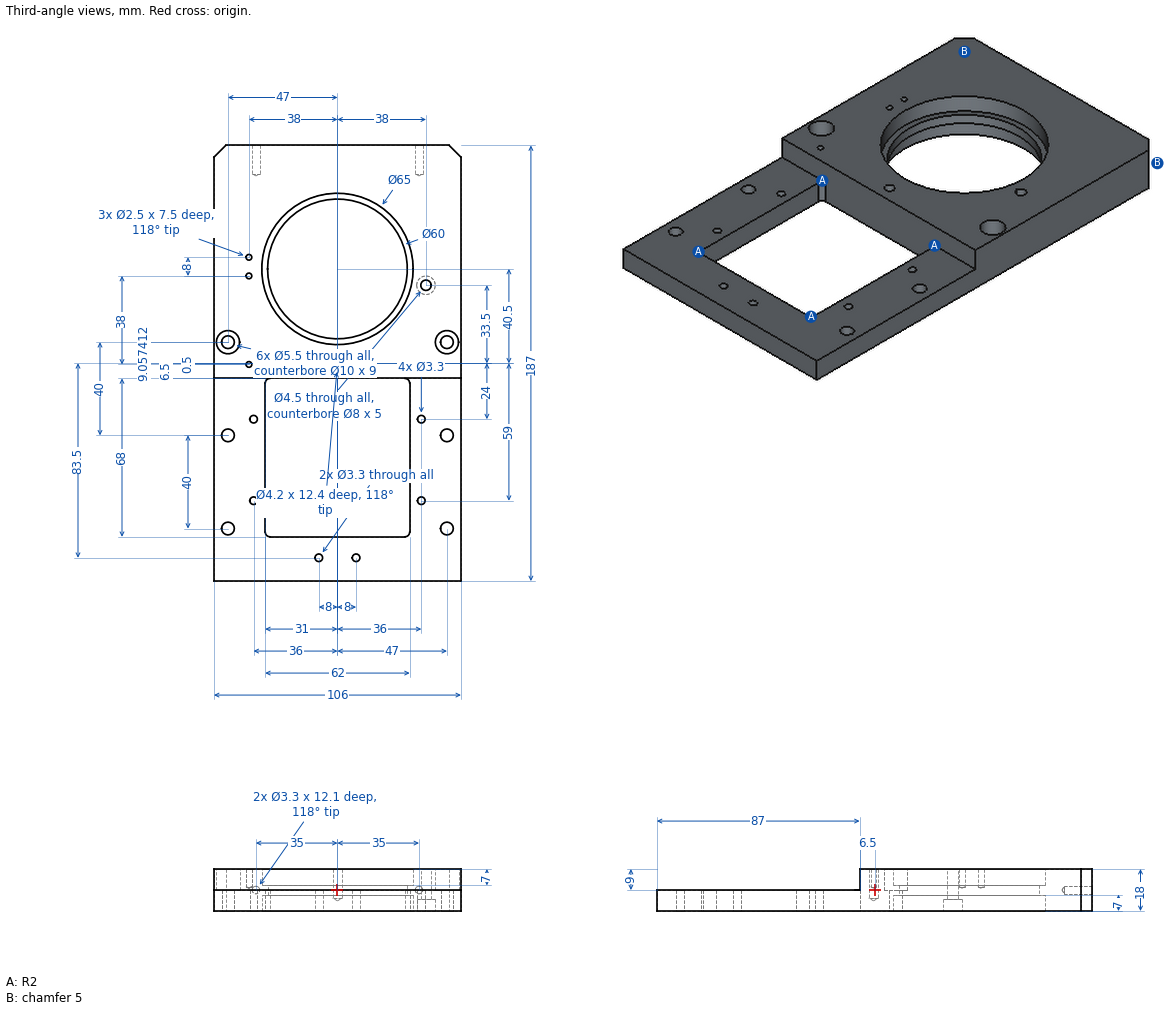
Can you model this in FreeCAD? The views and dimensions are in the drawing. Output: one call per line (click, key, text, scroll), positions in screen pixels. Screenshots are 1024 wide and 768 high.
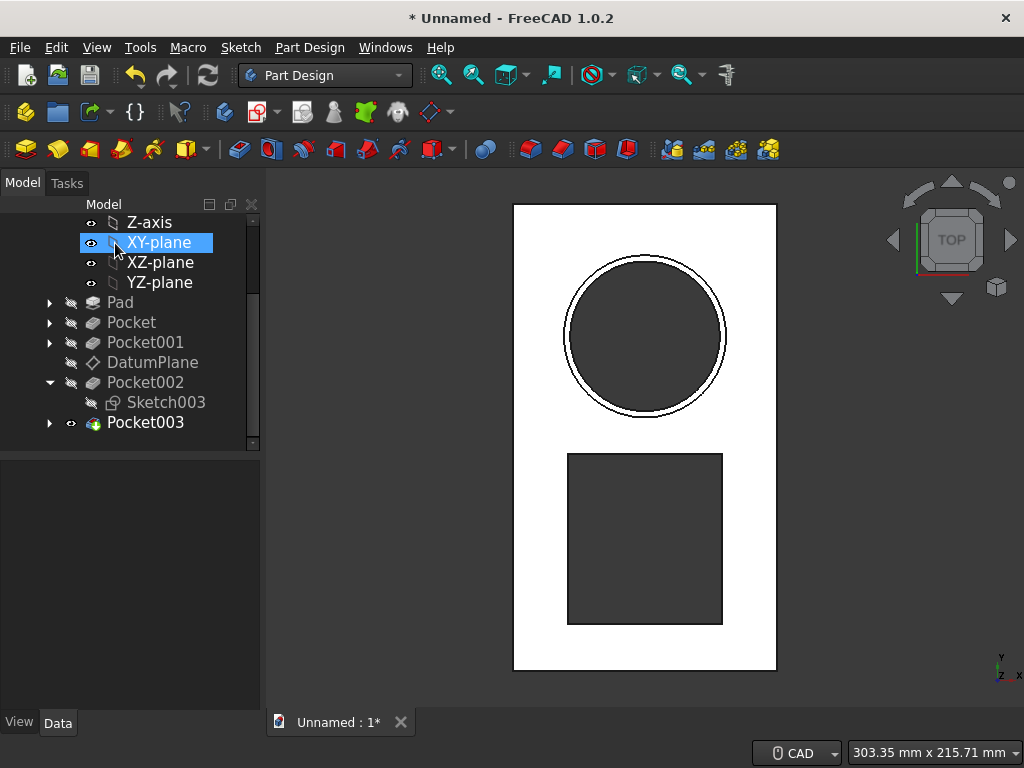
key(0)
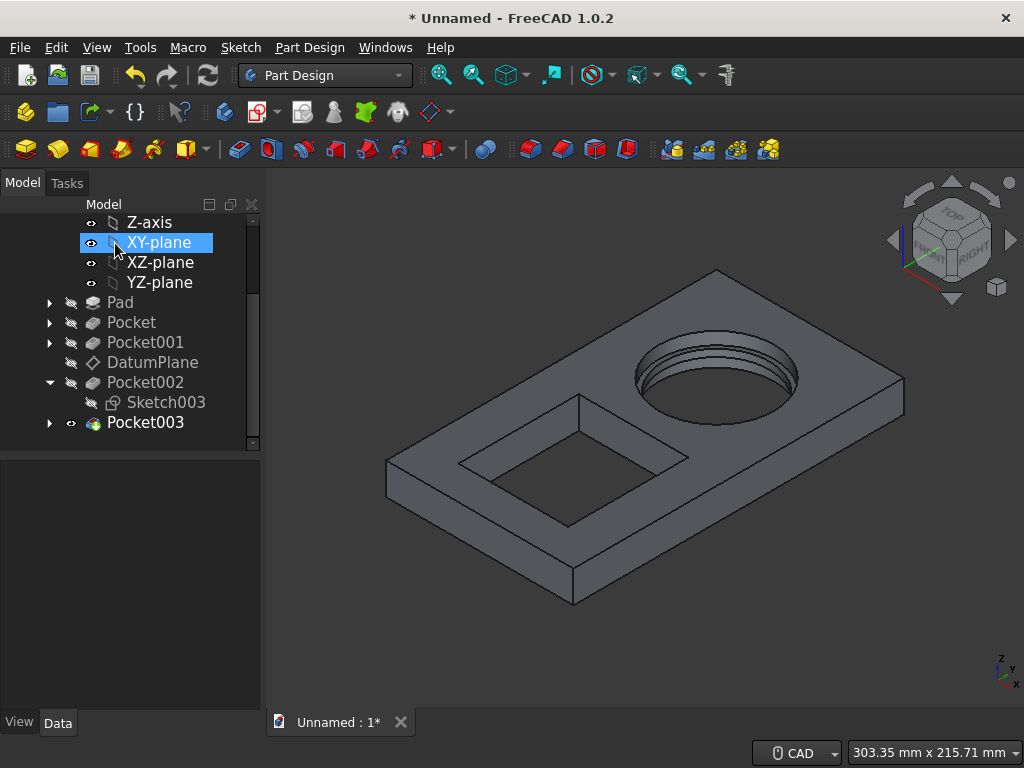
key(1)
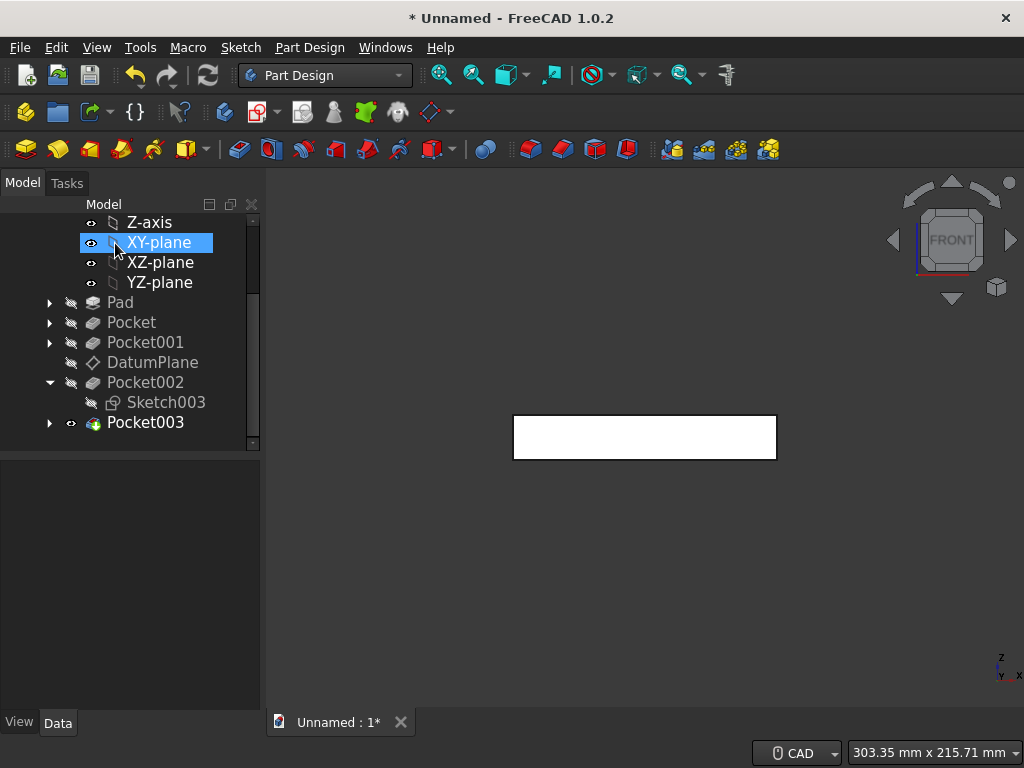
click(442, 76)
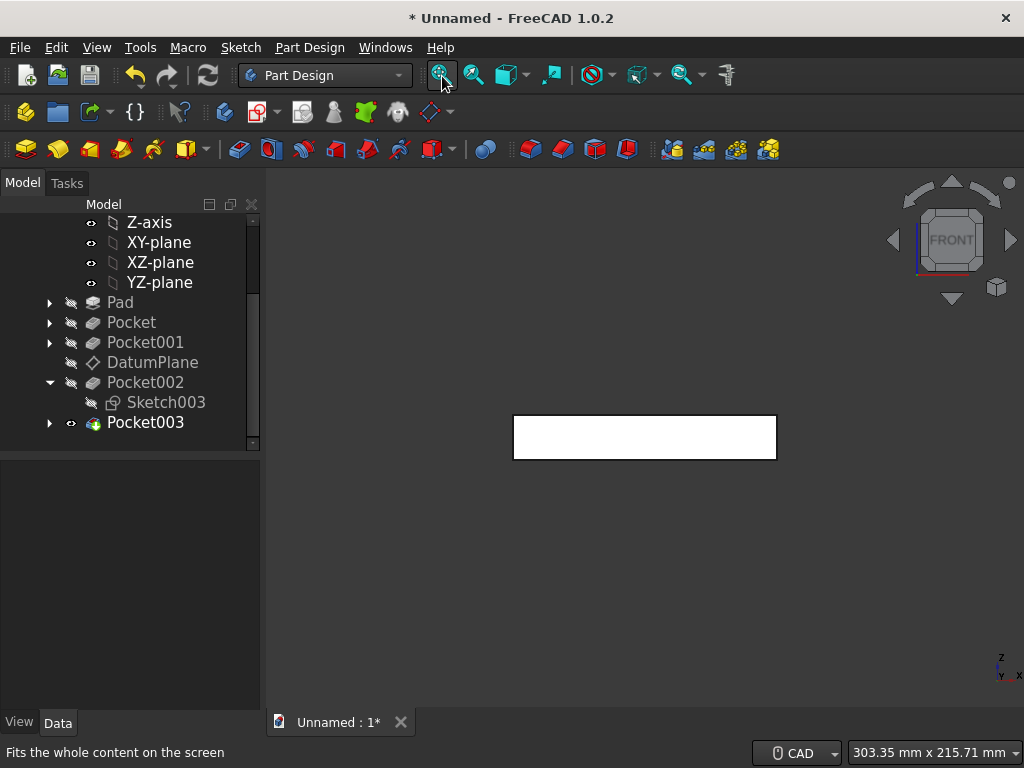
key(3)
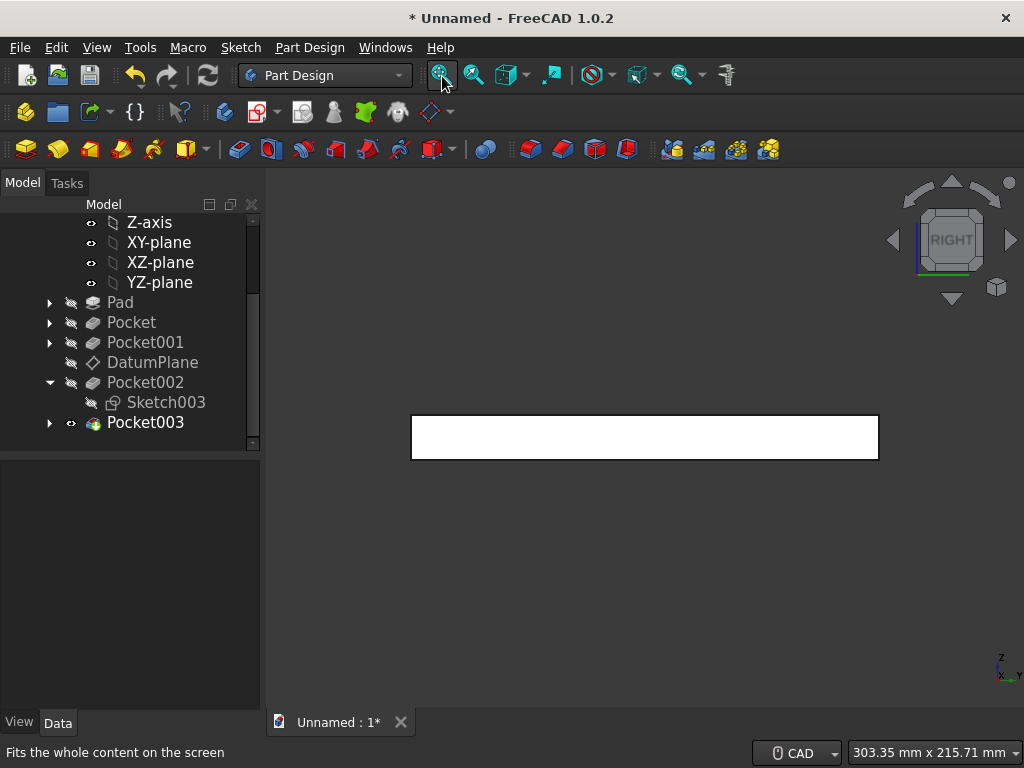
key(5)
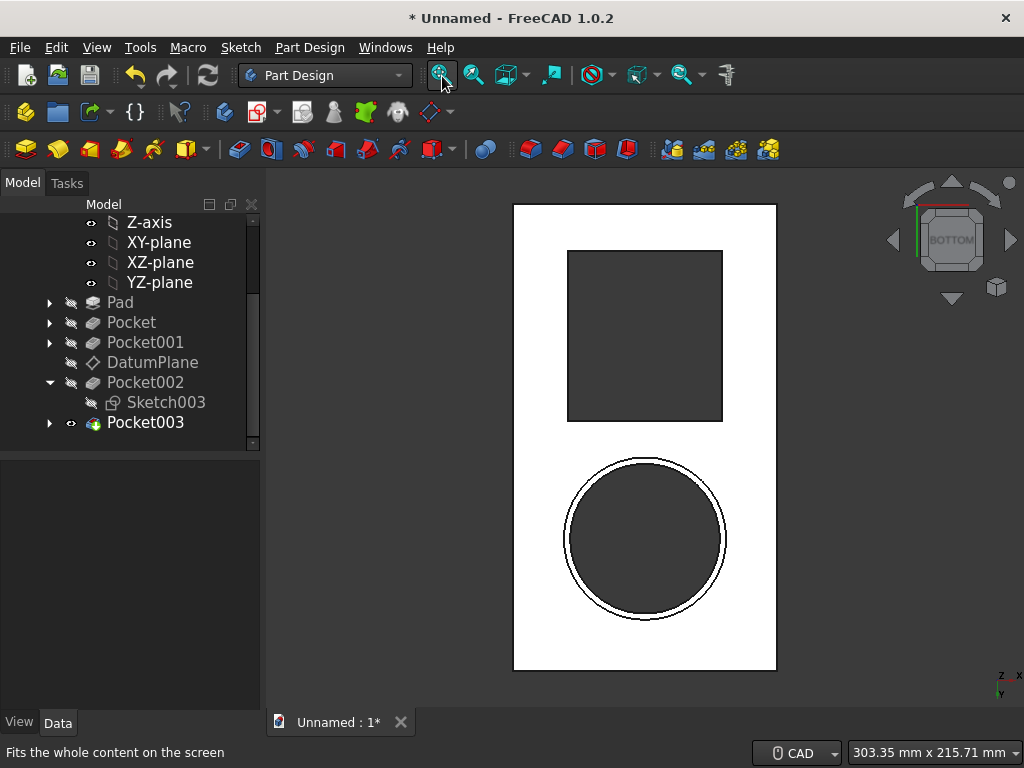
key(4)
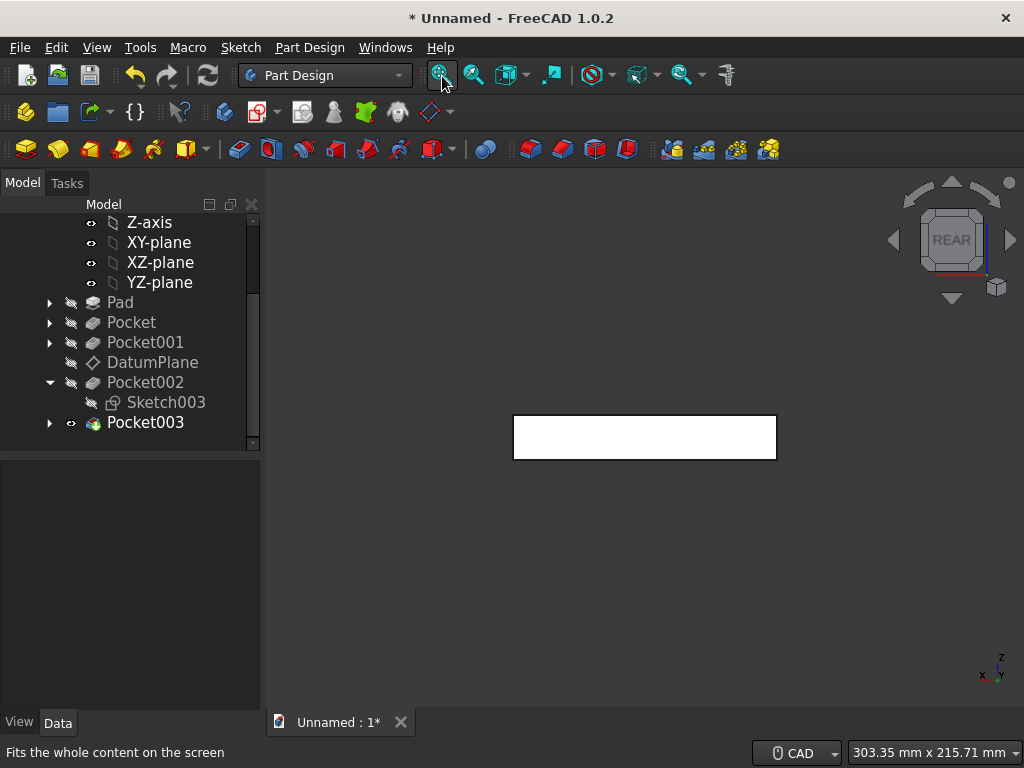
click(442, 76)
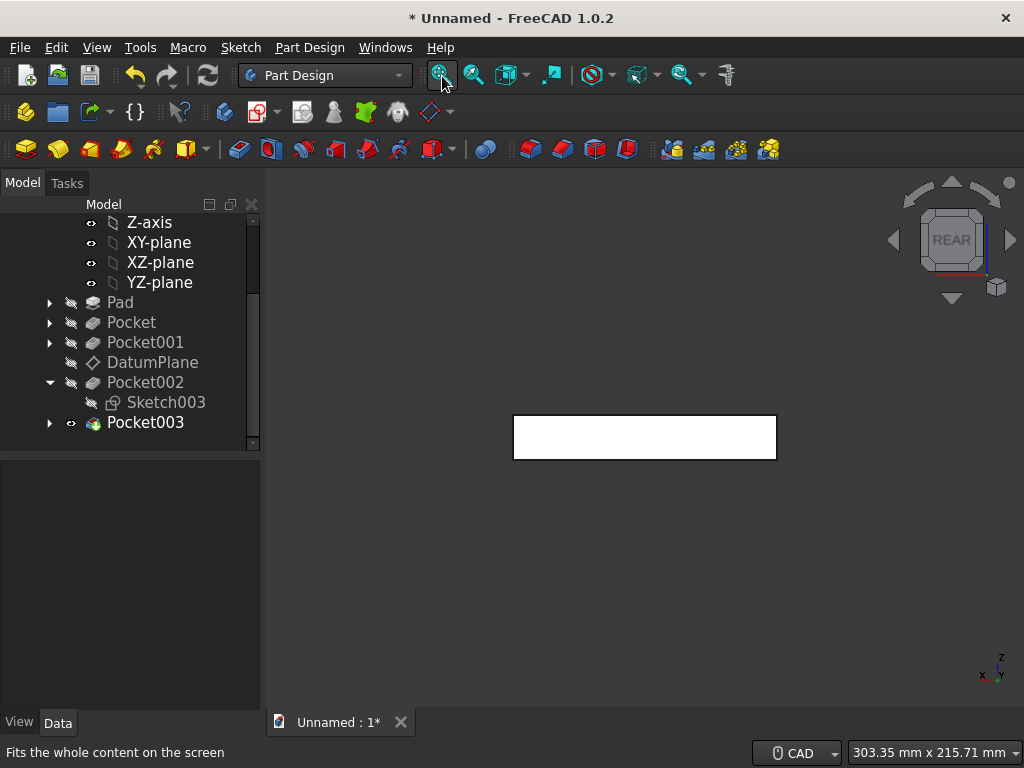
key(6)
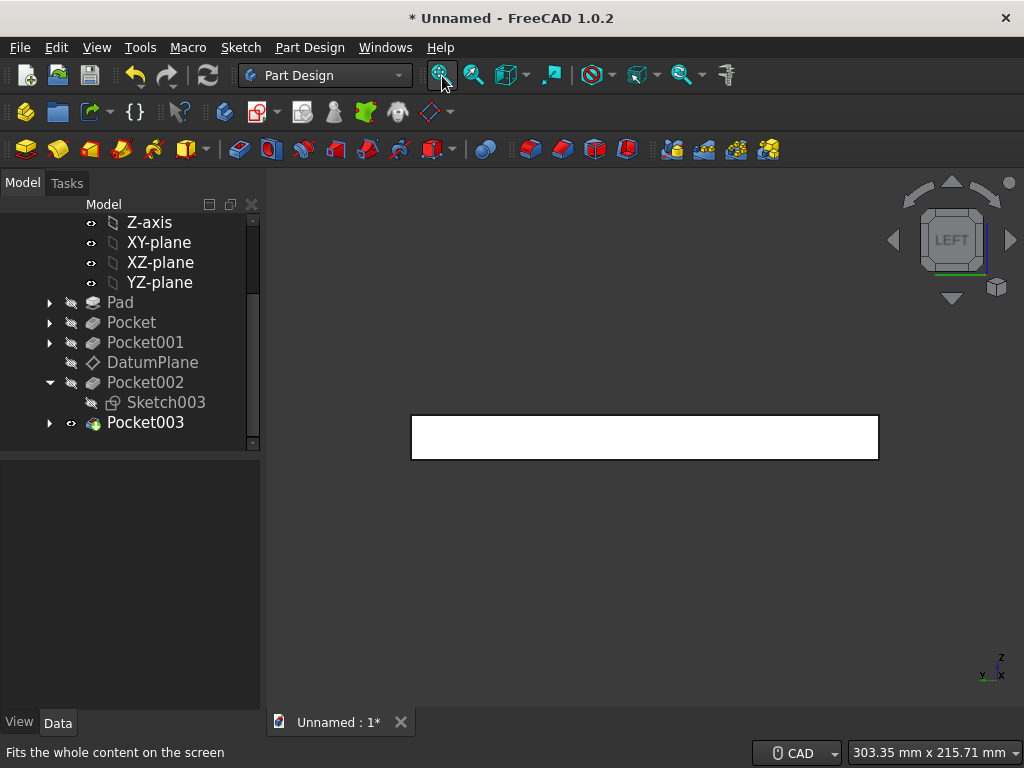
key(v)
key(3)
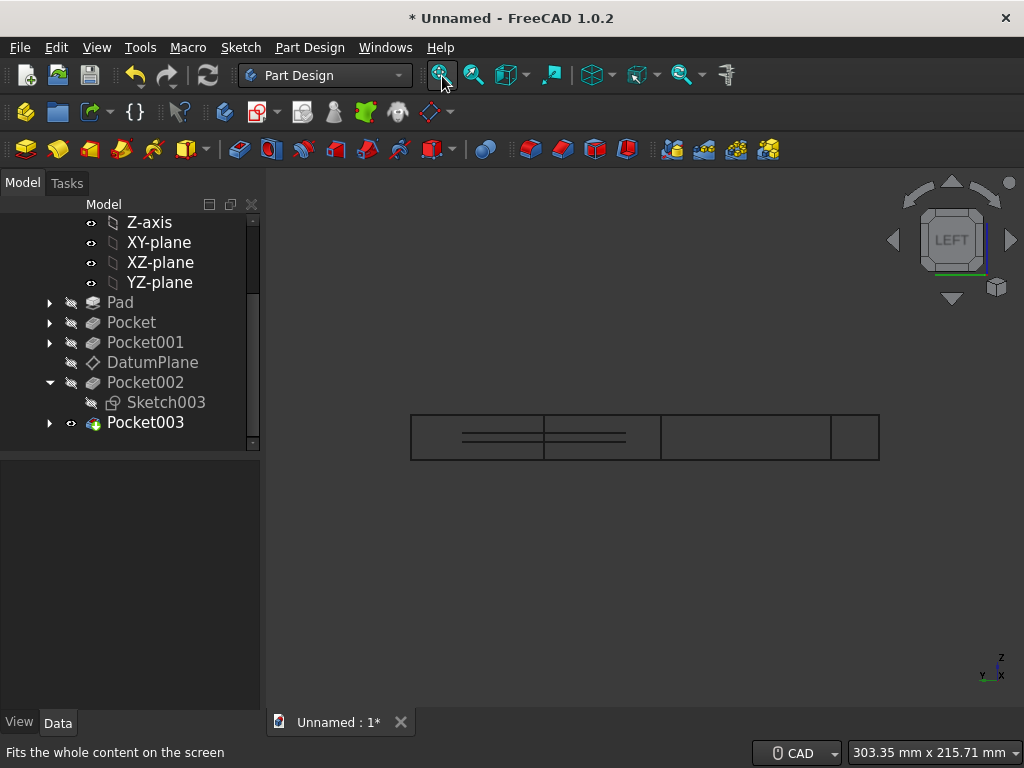
key(0)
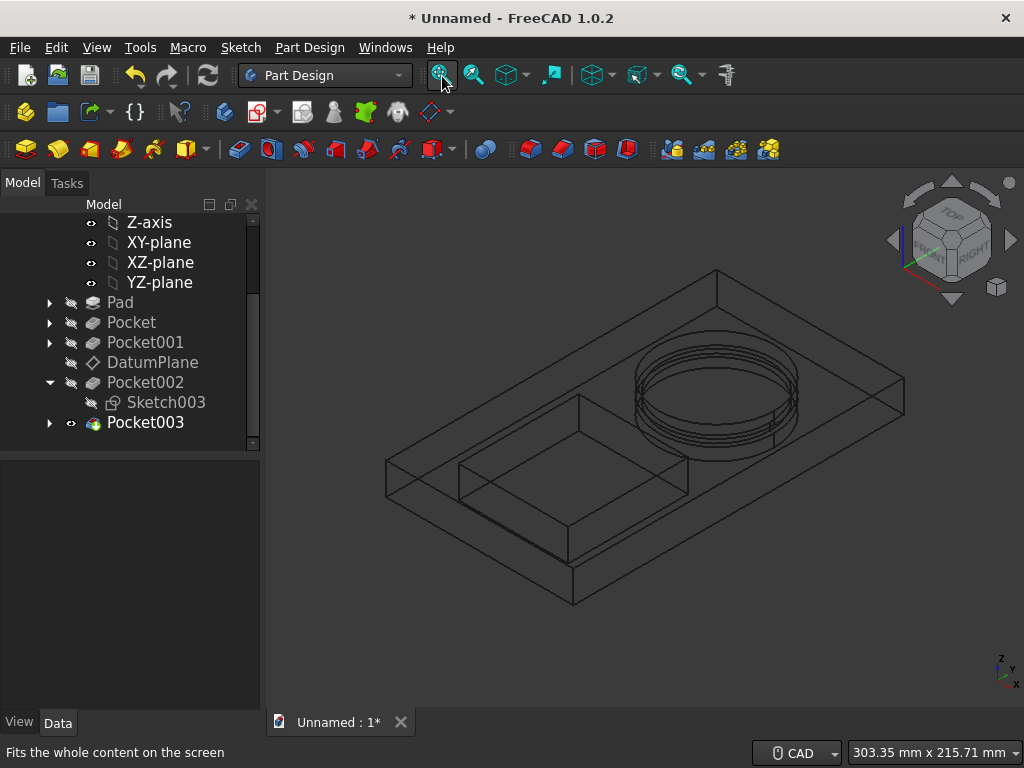
click(459, 481)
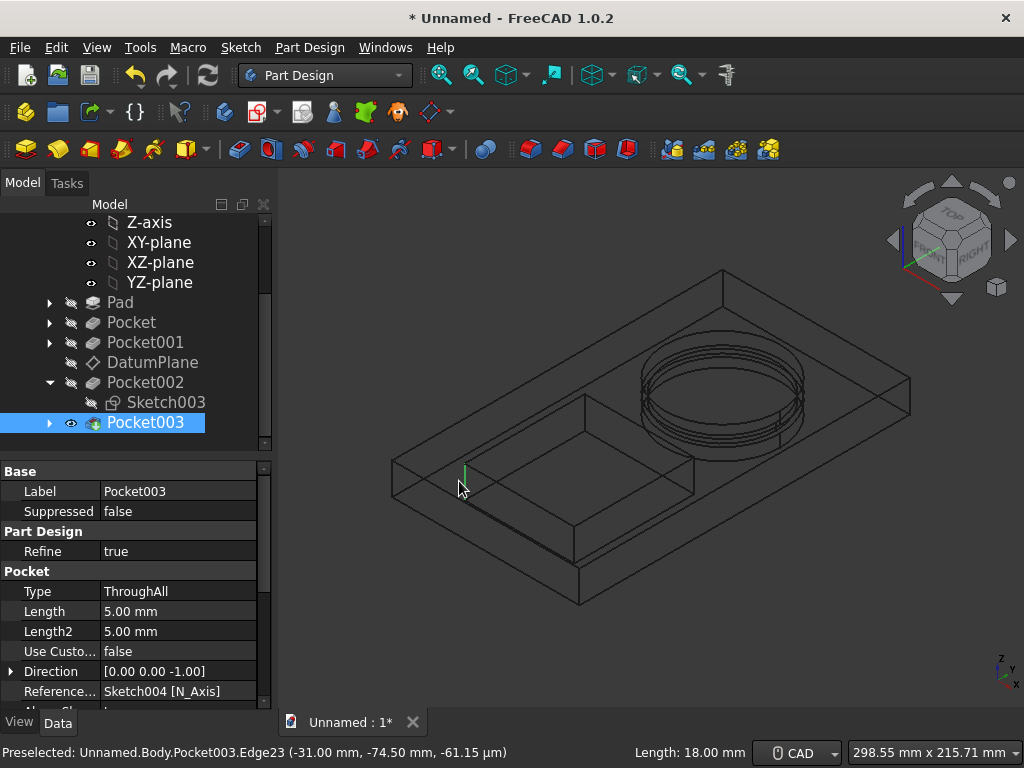
click(585, 412, ctrl)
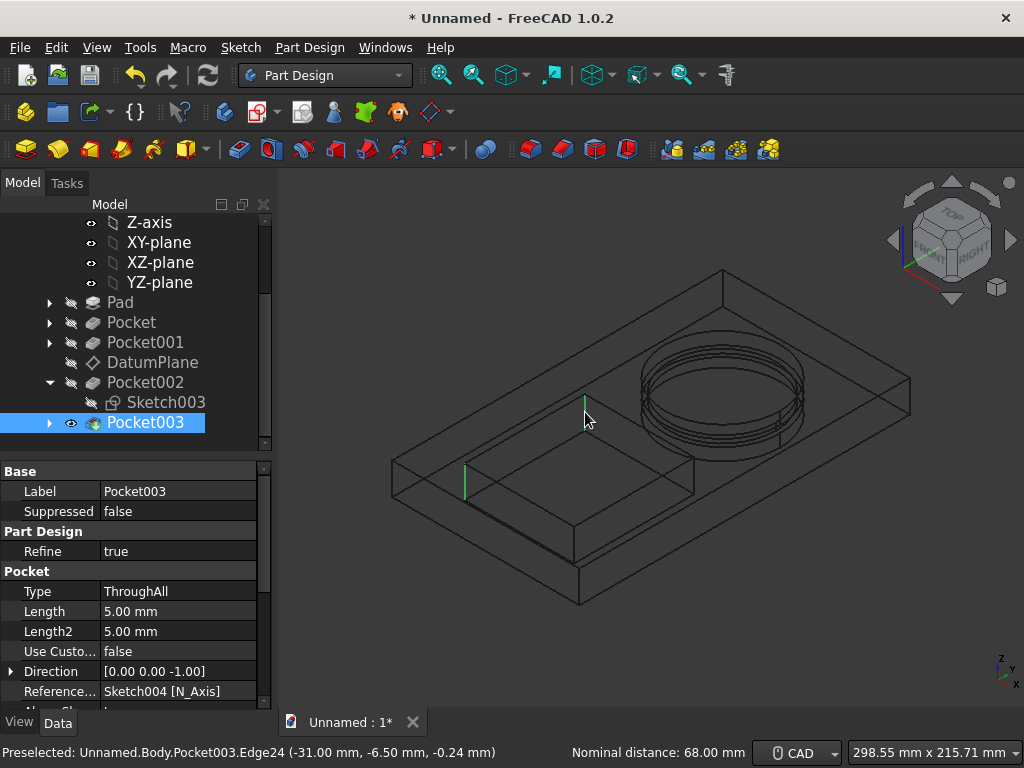
click(694, 475, ctrl)